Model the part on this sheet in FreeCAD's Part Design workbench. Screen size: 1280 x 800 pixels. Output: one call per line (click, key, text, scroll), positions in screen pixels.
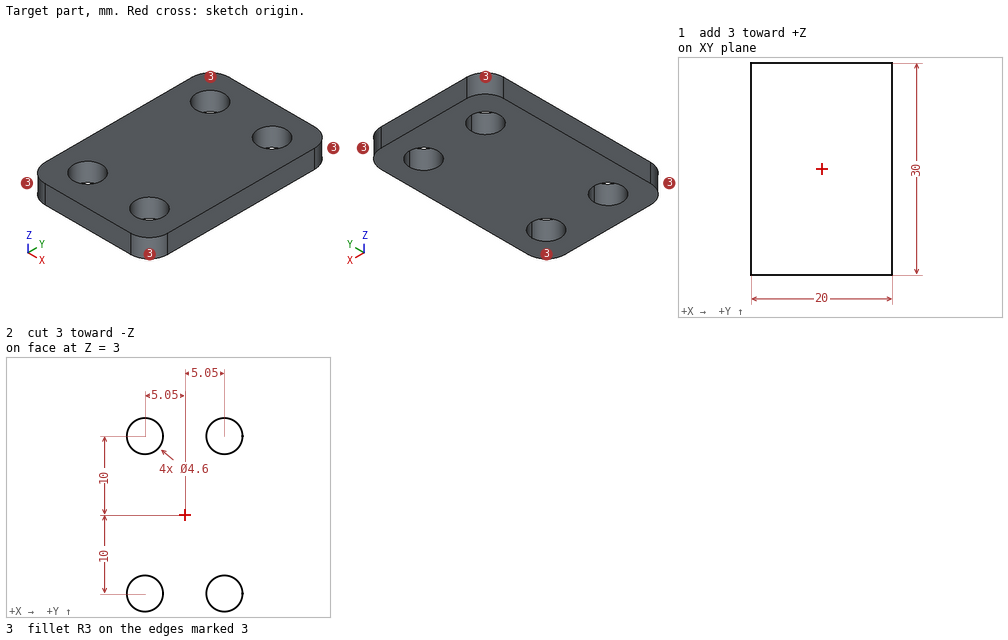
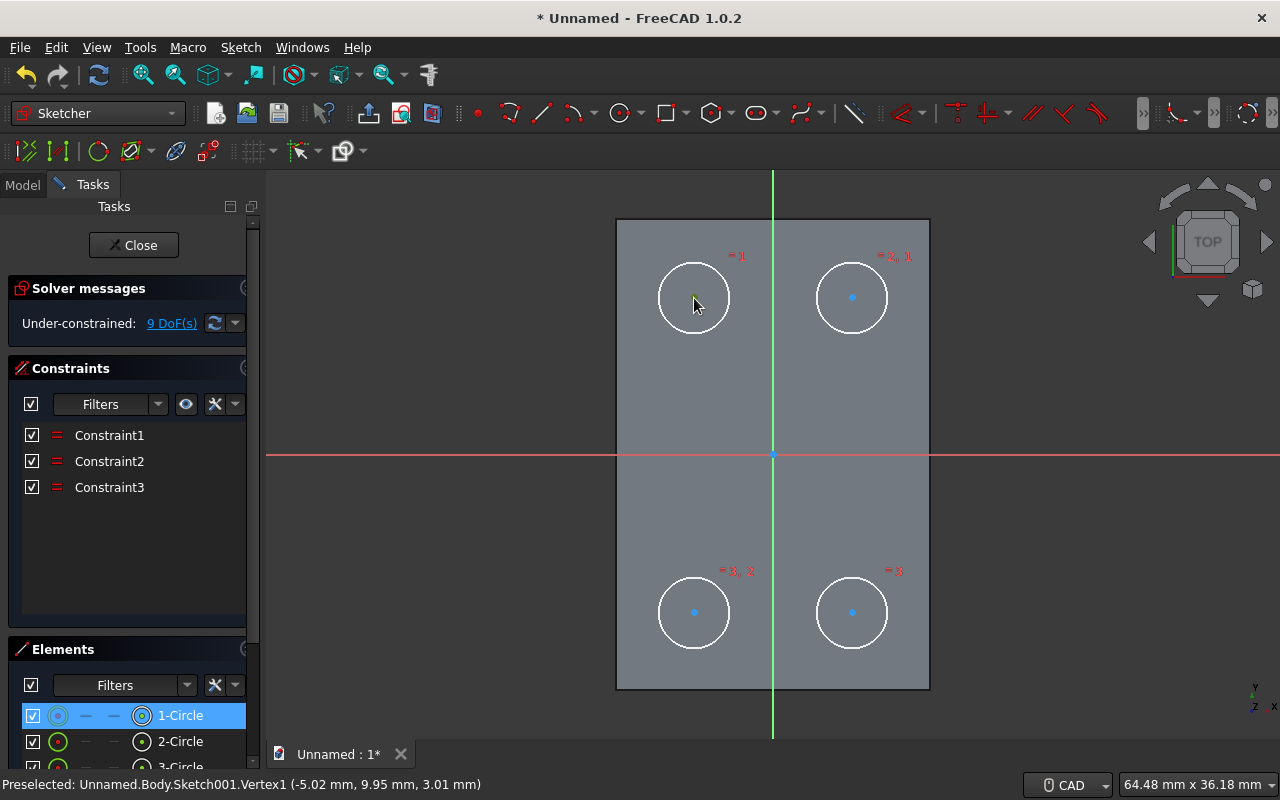
click(852, 298)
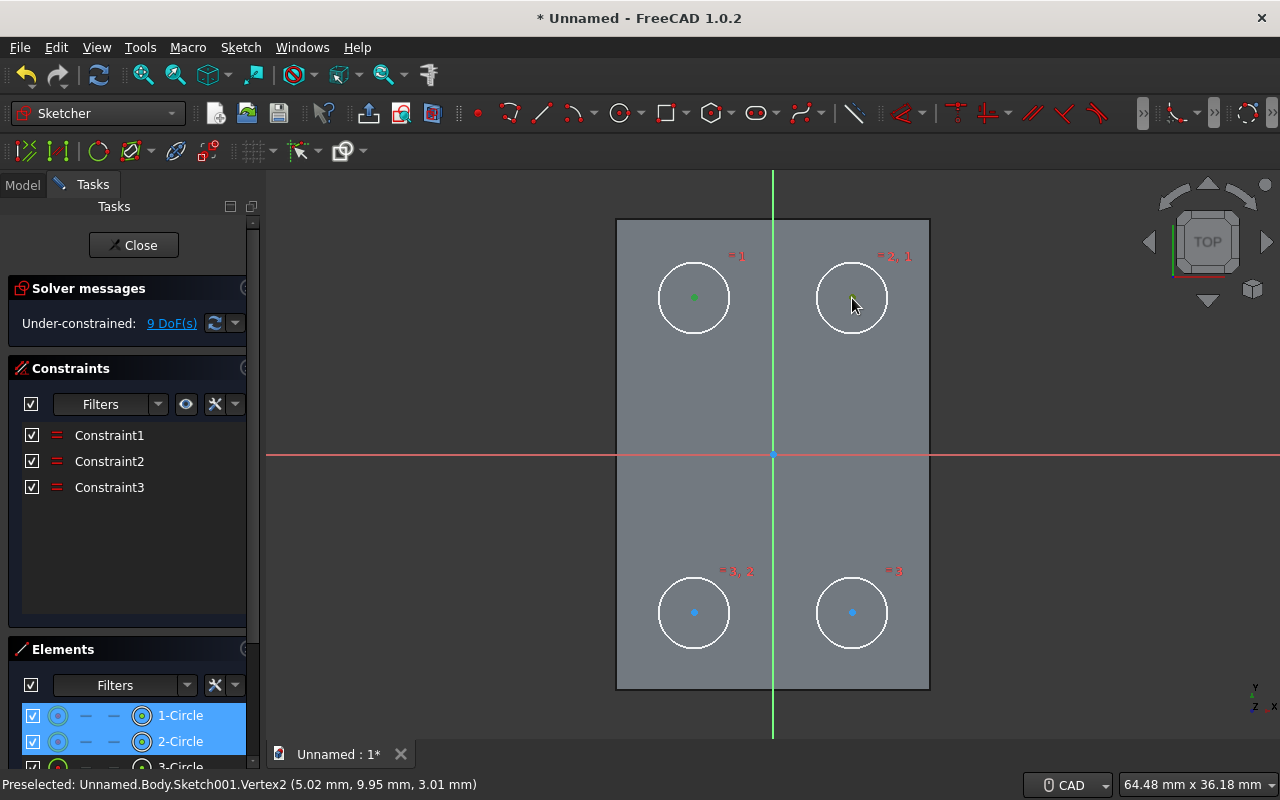
key(h)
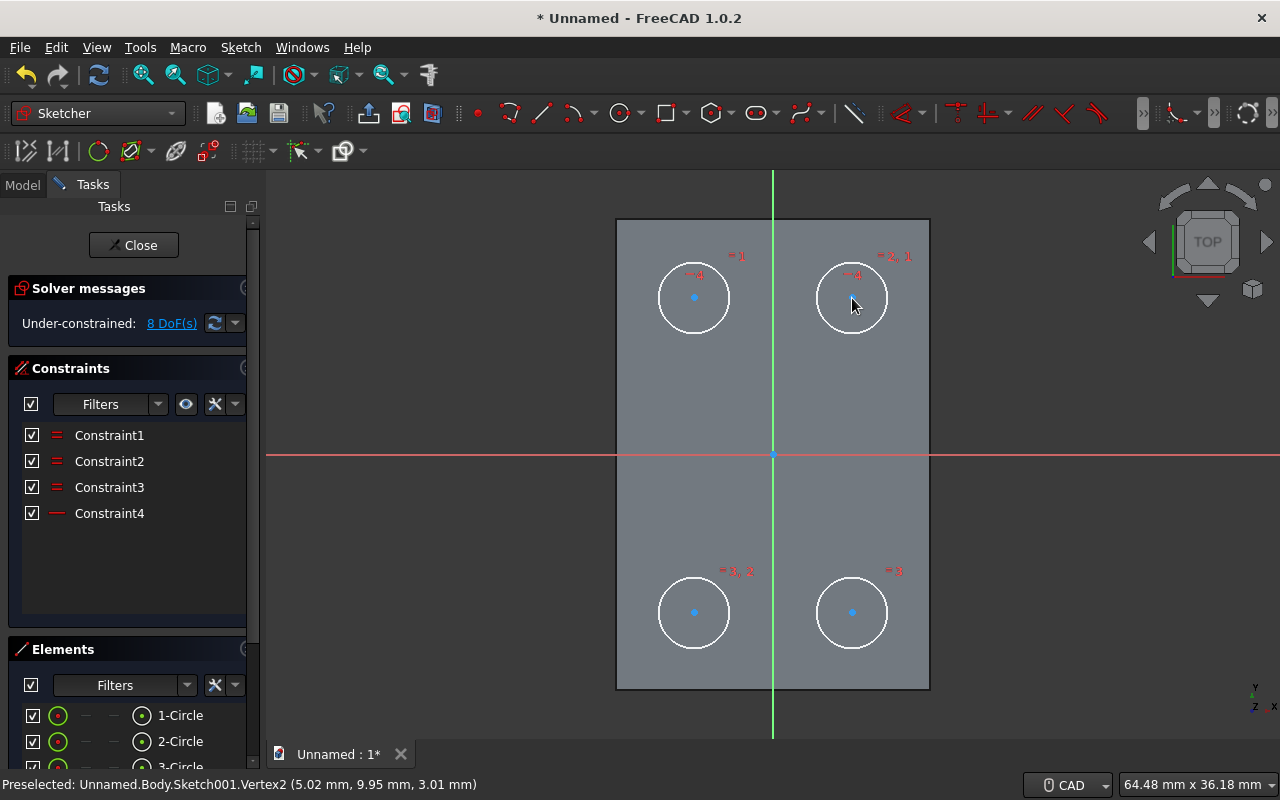
click(694, 298)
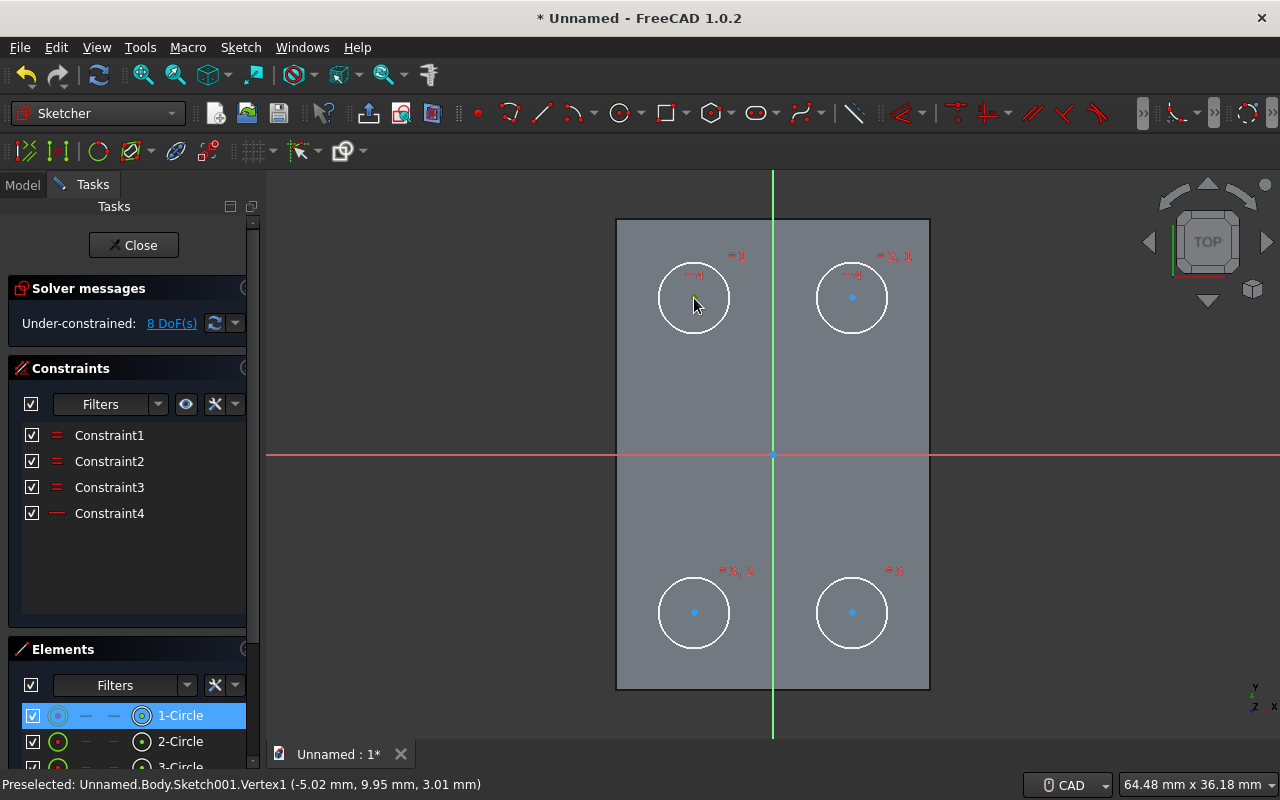
click(694, 613)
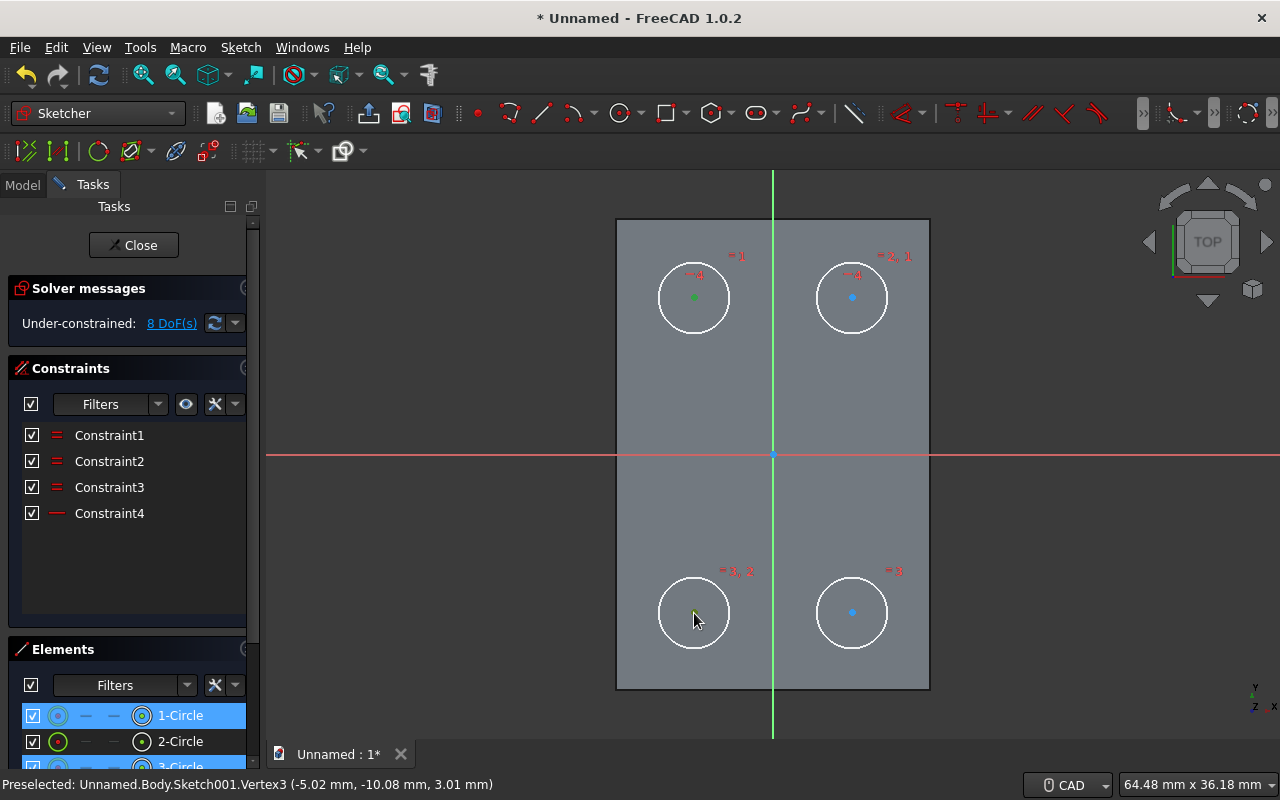
click(1010, 114)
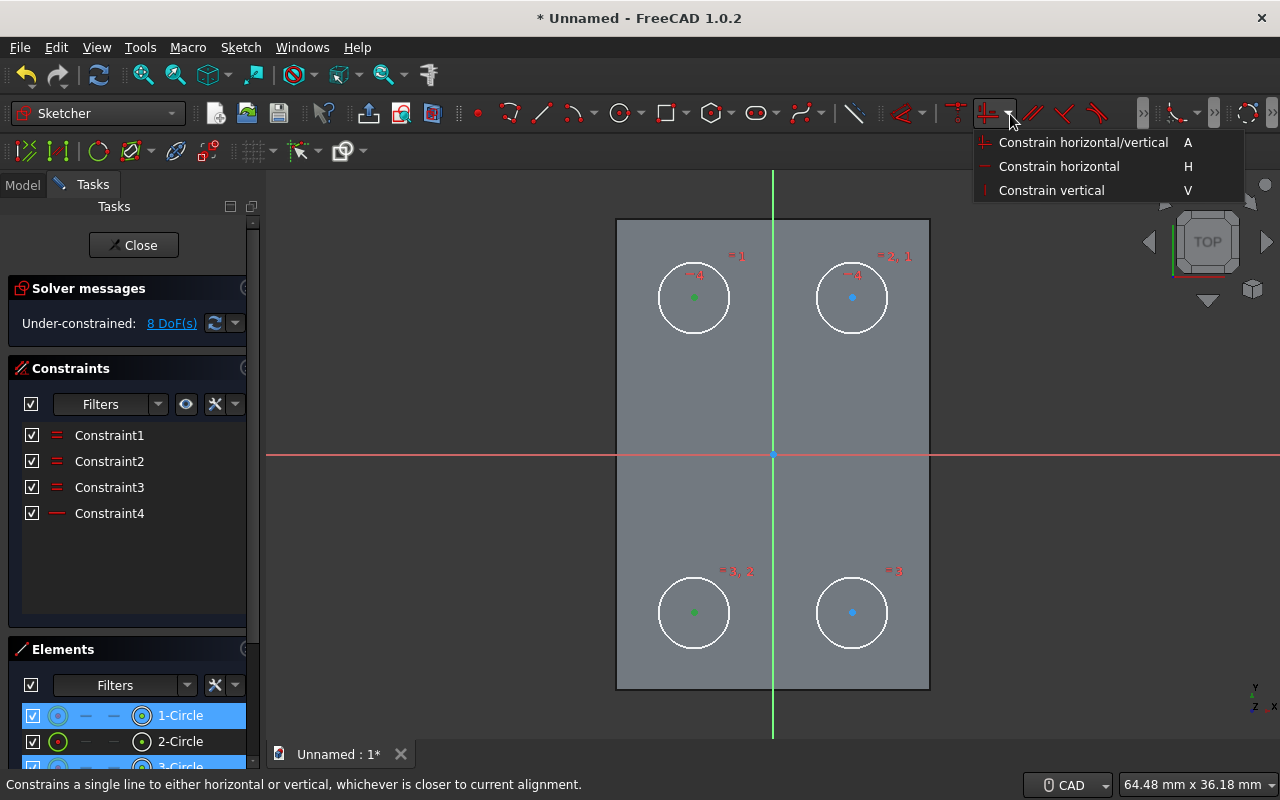
click(1109, 190)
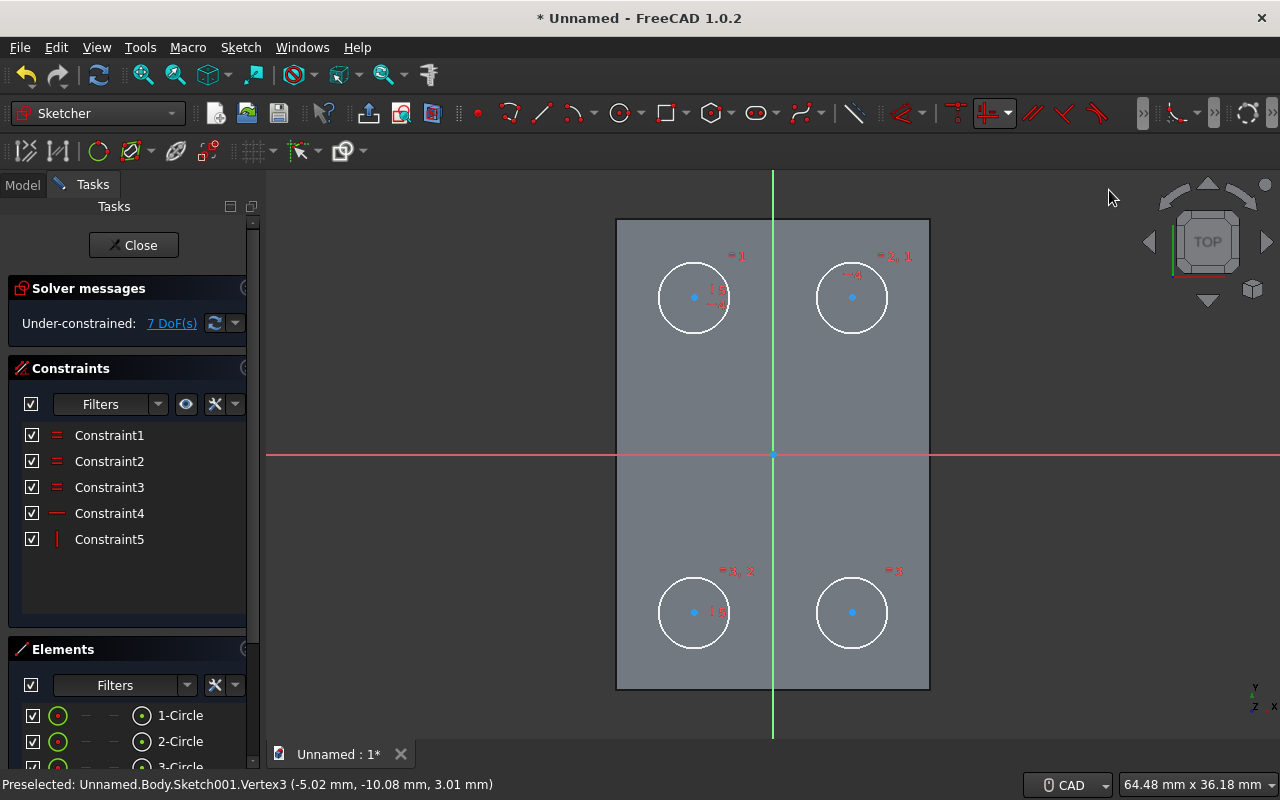
click(852, 298)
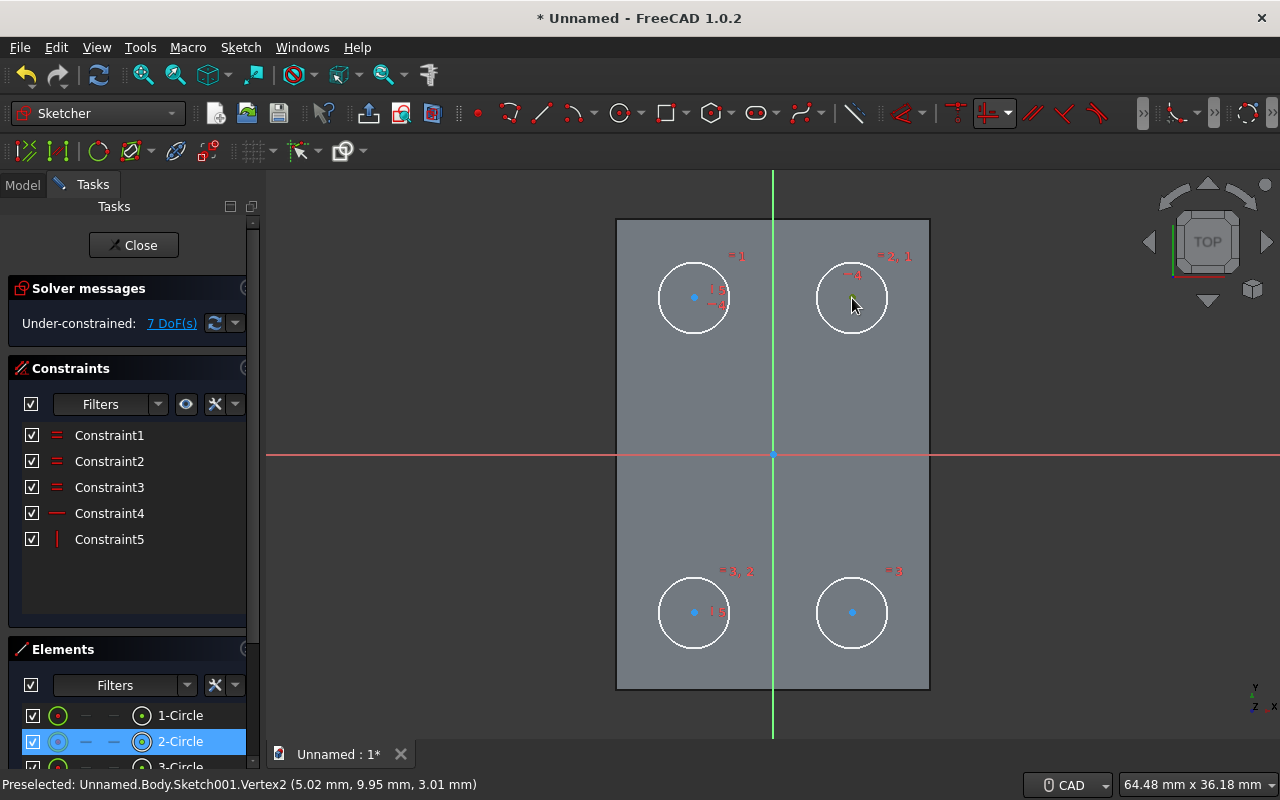
click(852, 613)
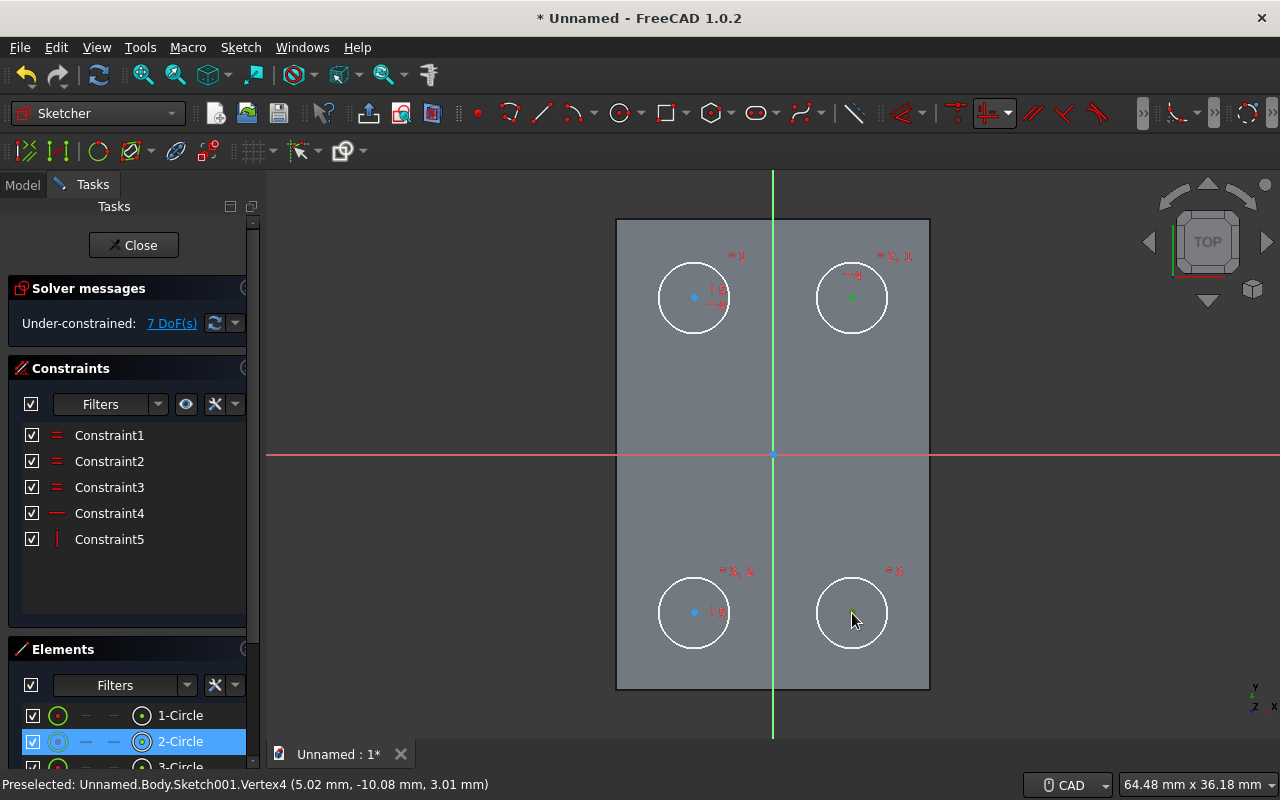
key(v)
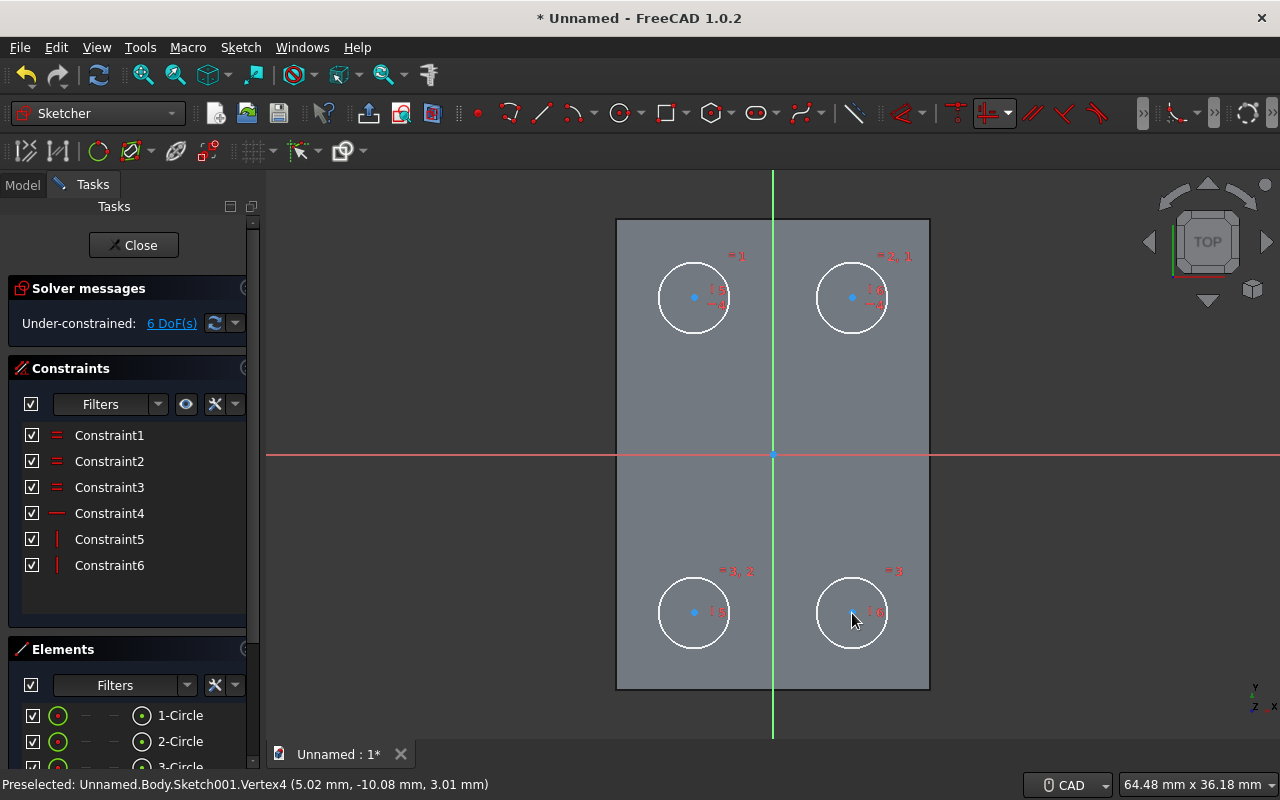
click(694, 613)